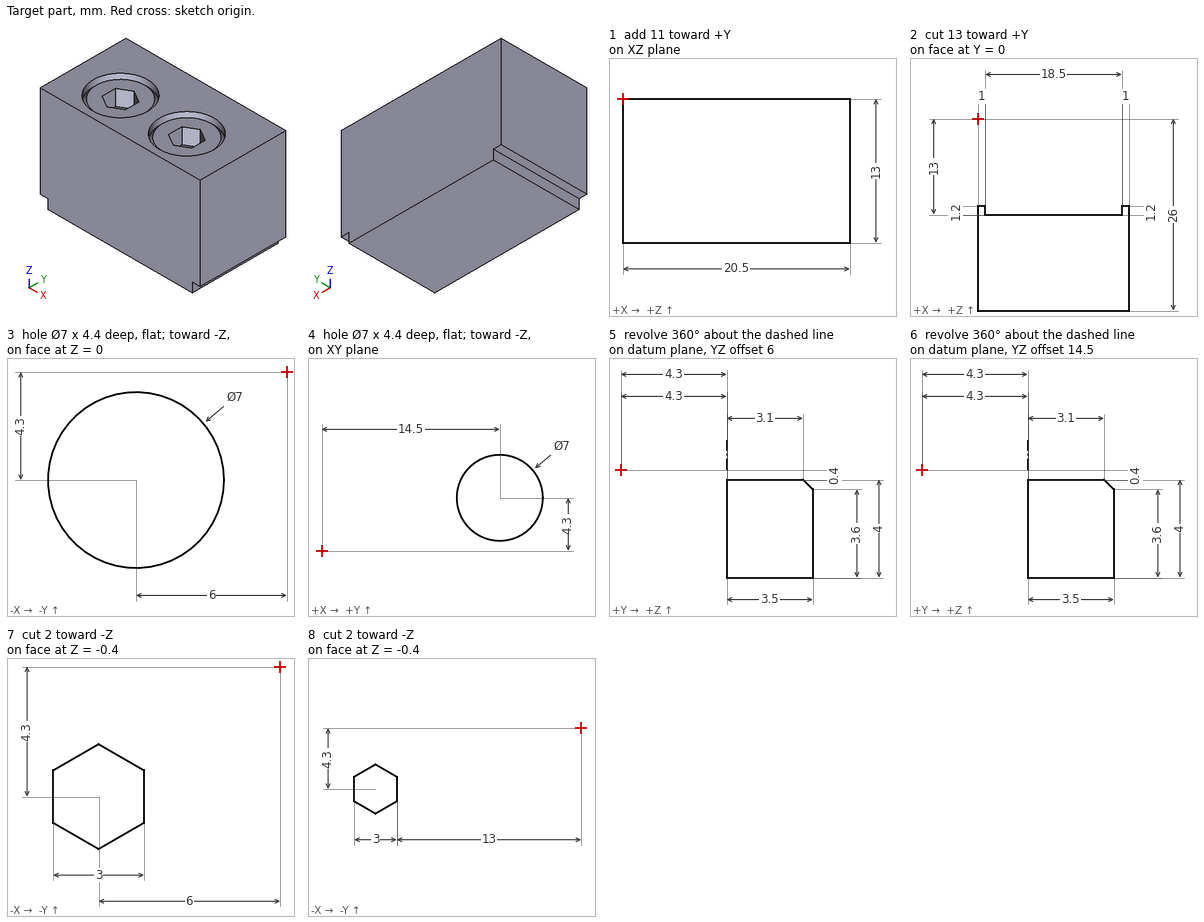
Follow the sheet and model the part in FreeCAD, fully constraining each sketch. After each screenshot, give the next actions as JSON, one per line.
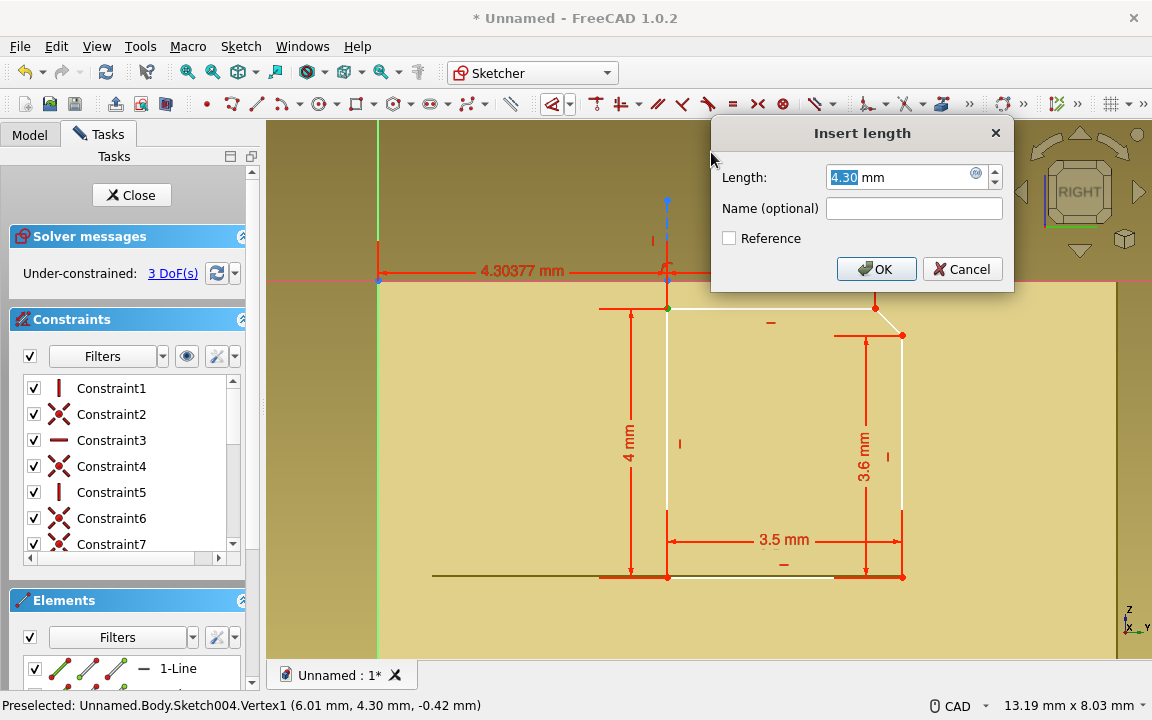
{"action": "type", "text": "4.3"}
{"action": "key", "text": "Return"}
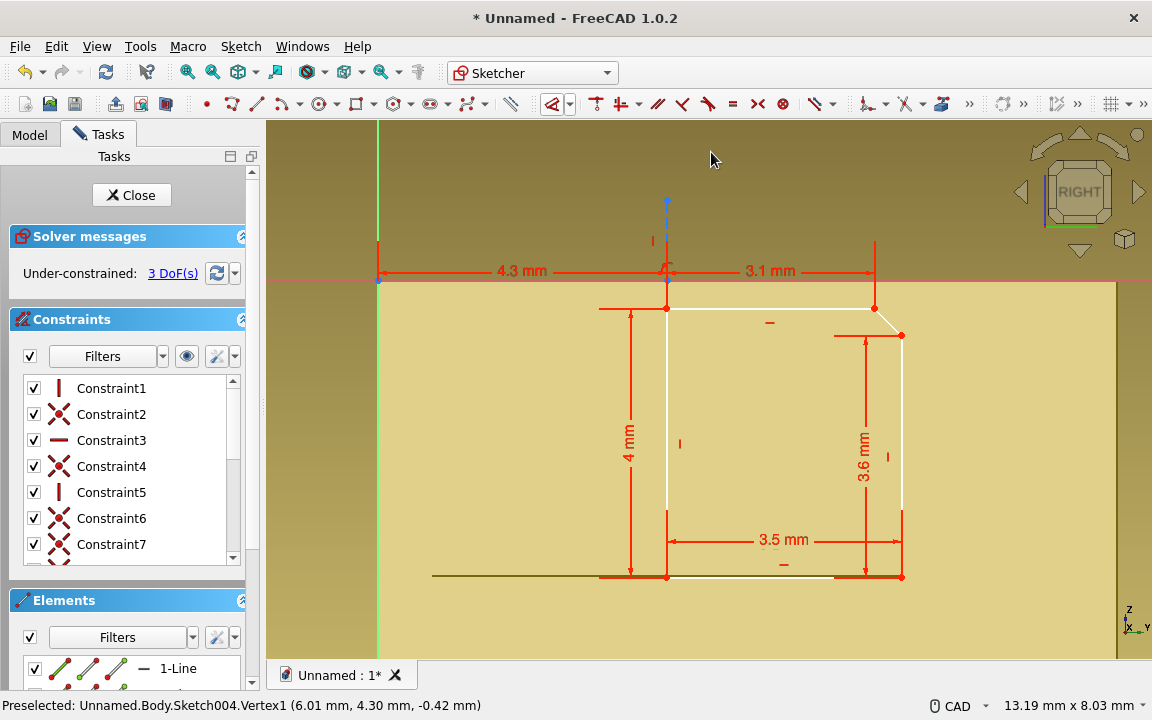
{"action": "scroll", "coordinate": [667, 309], "scroll_direction": "up", "scroll_amount": 2}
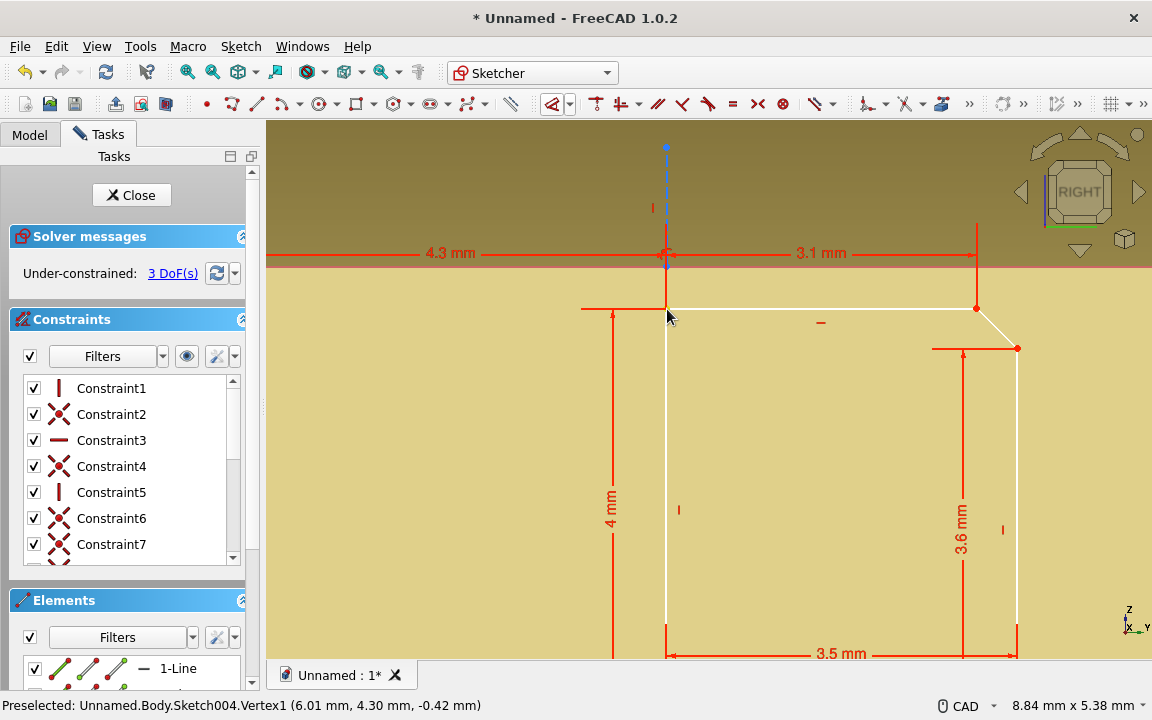
{"action": "left_click", "coordinate": [666, 309]}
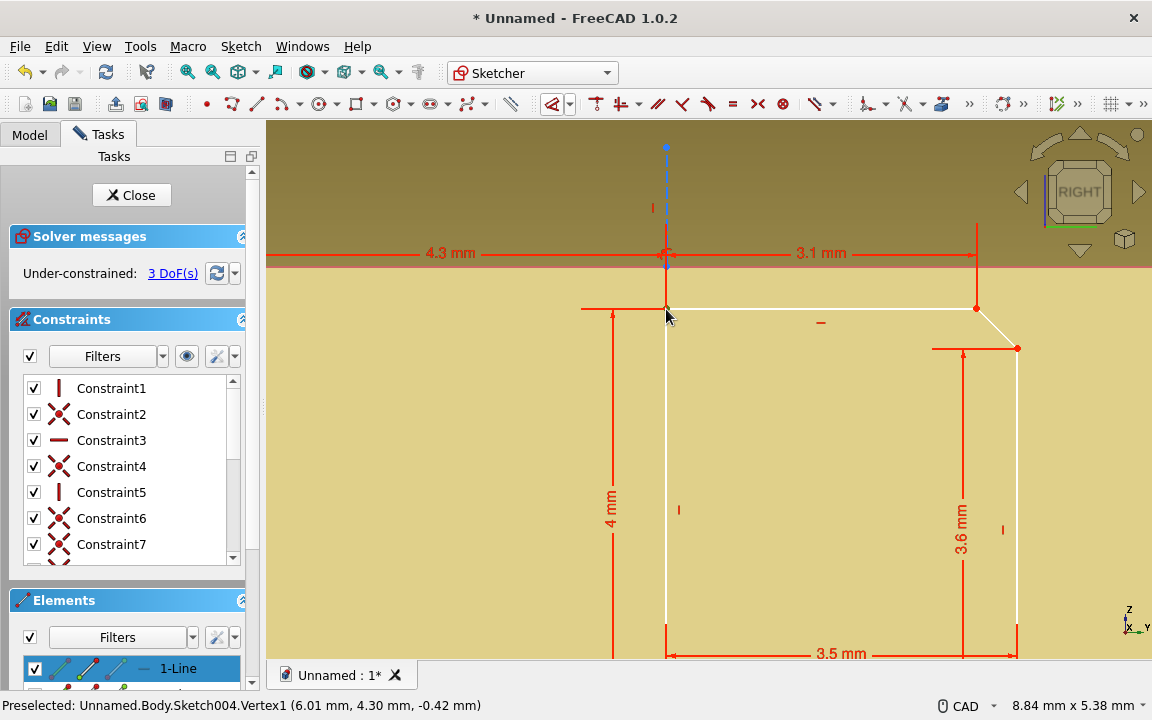
{"action": "left_click", "coordinate": [570, 104]}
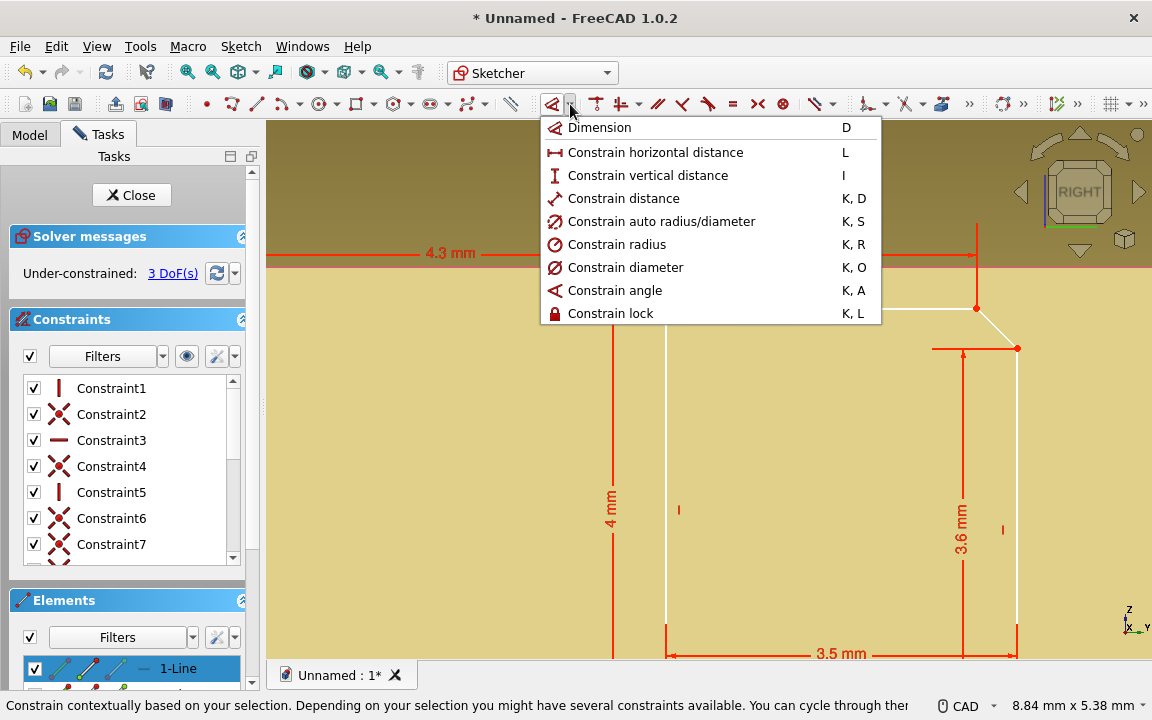
{"action": "left_click", "coordinate": [711, 176]}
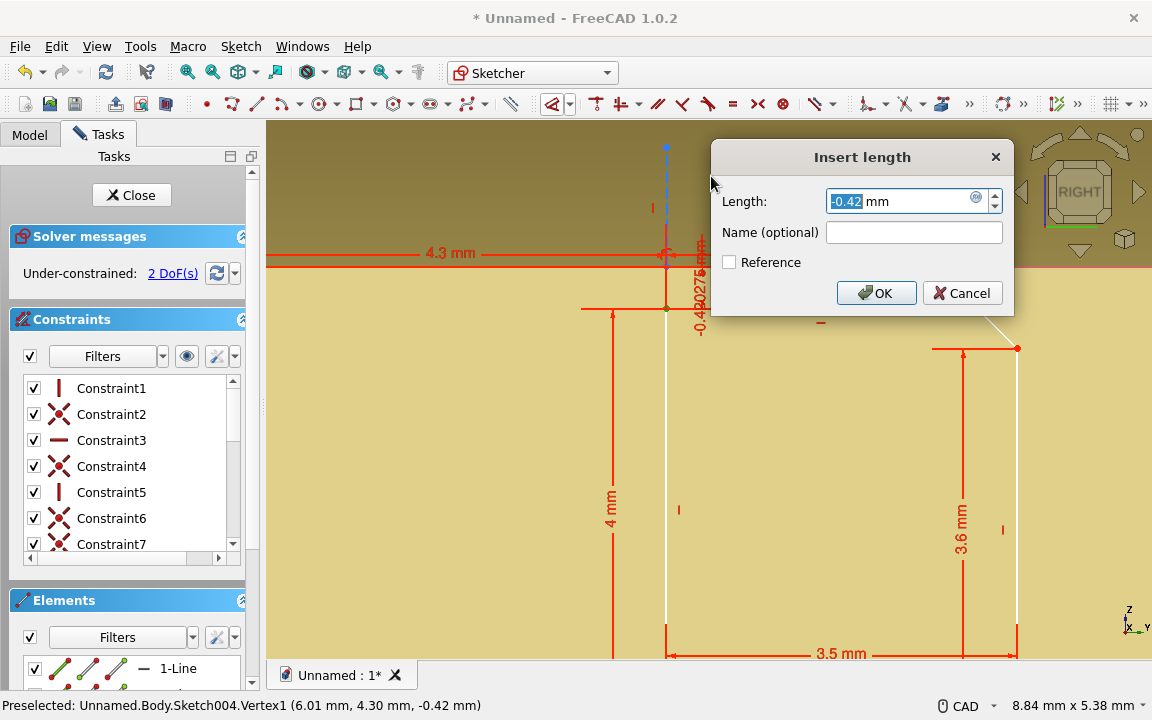
{"action": "type", "text": "-0.4"}
{"action": "key", "text": "Return"}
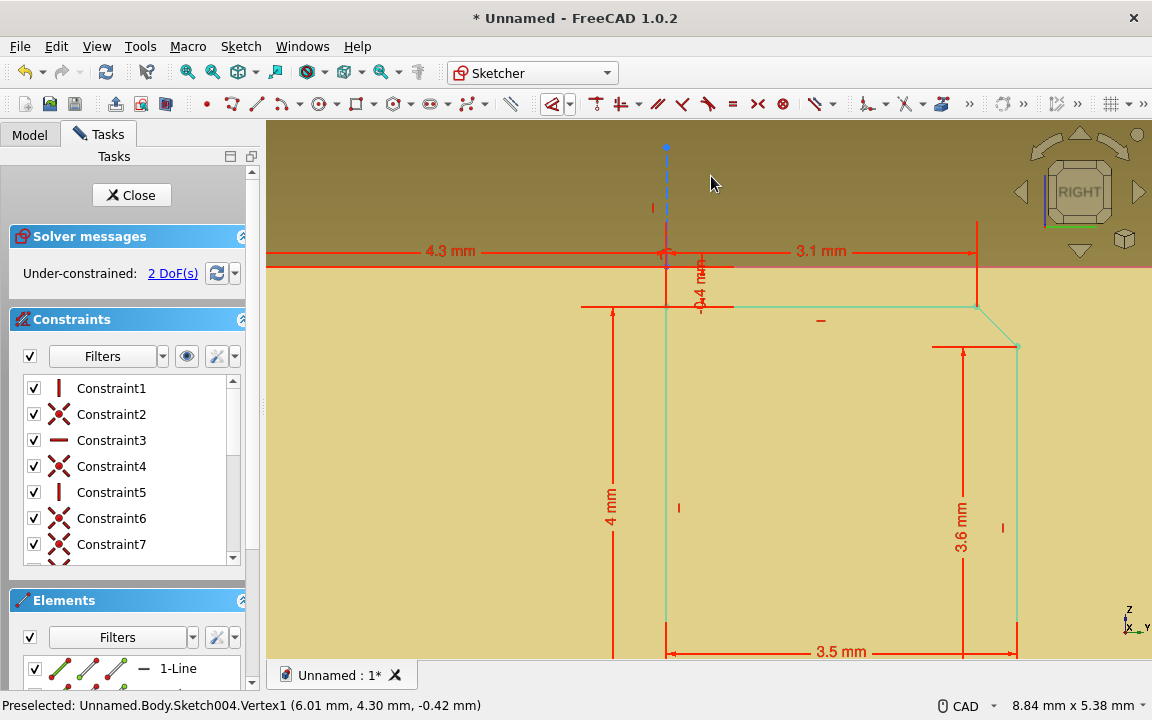
{"action": "left_click", "coordinate": [667, 267]}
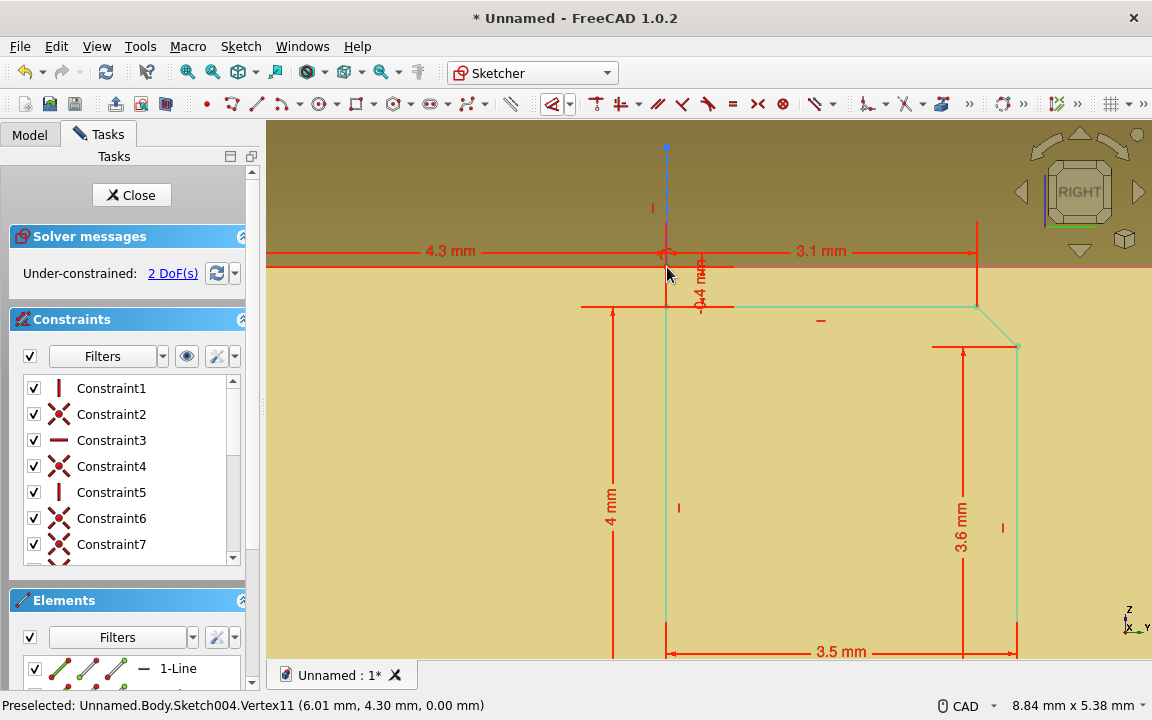
{"action": "key", "text": "l"}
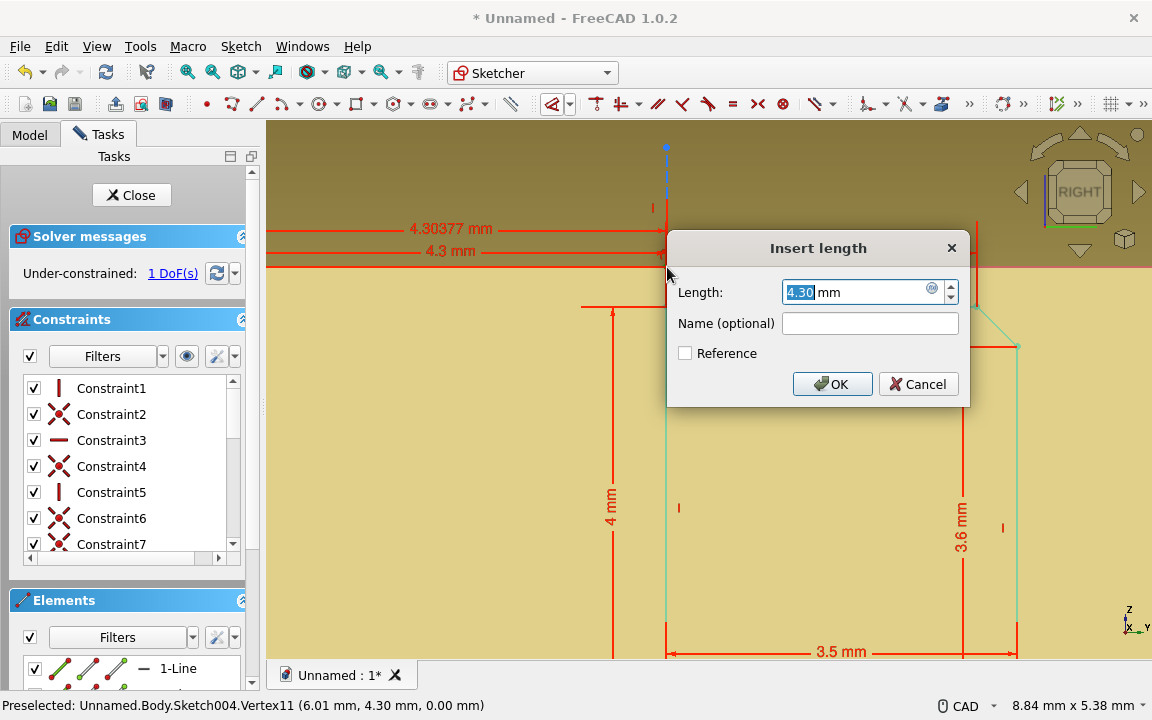
{"action": "type", "text": "4.3"}
{"action": "key", "text": "Return"}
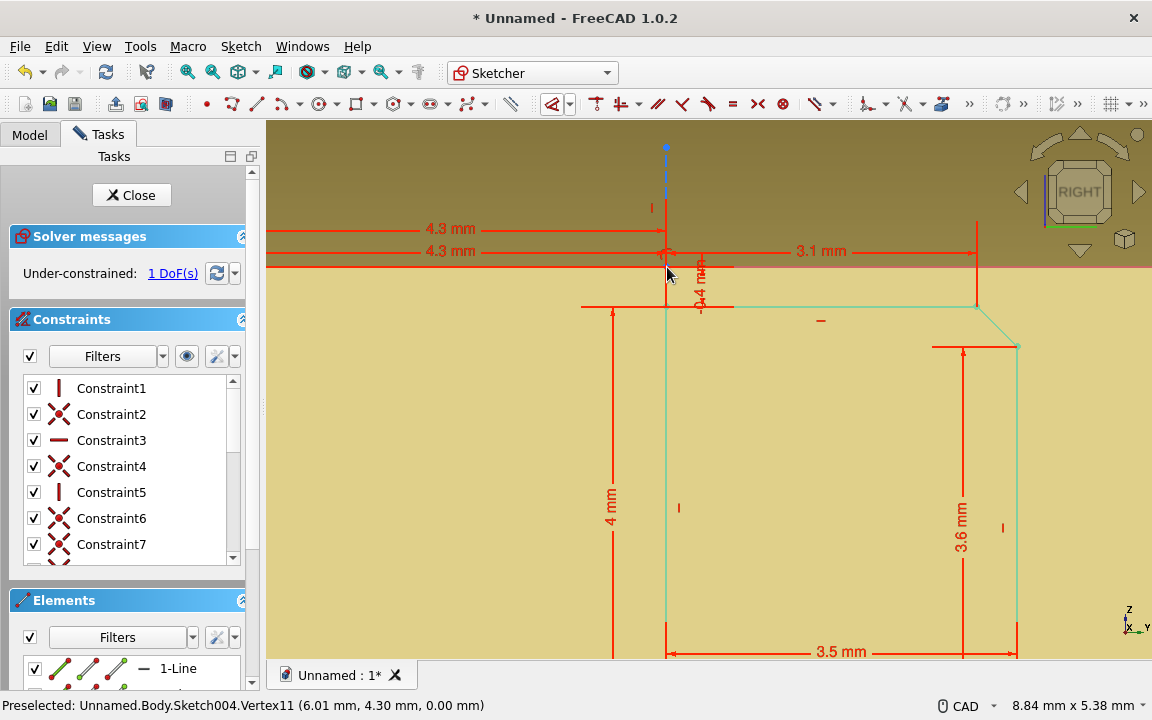
{"action": "left_click", "coordinate": [132, 195]}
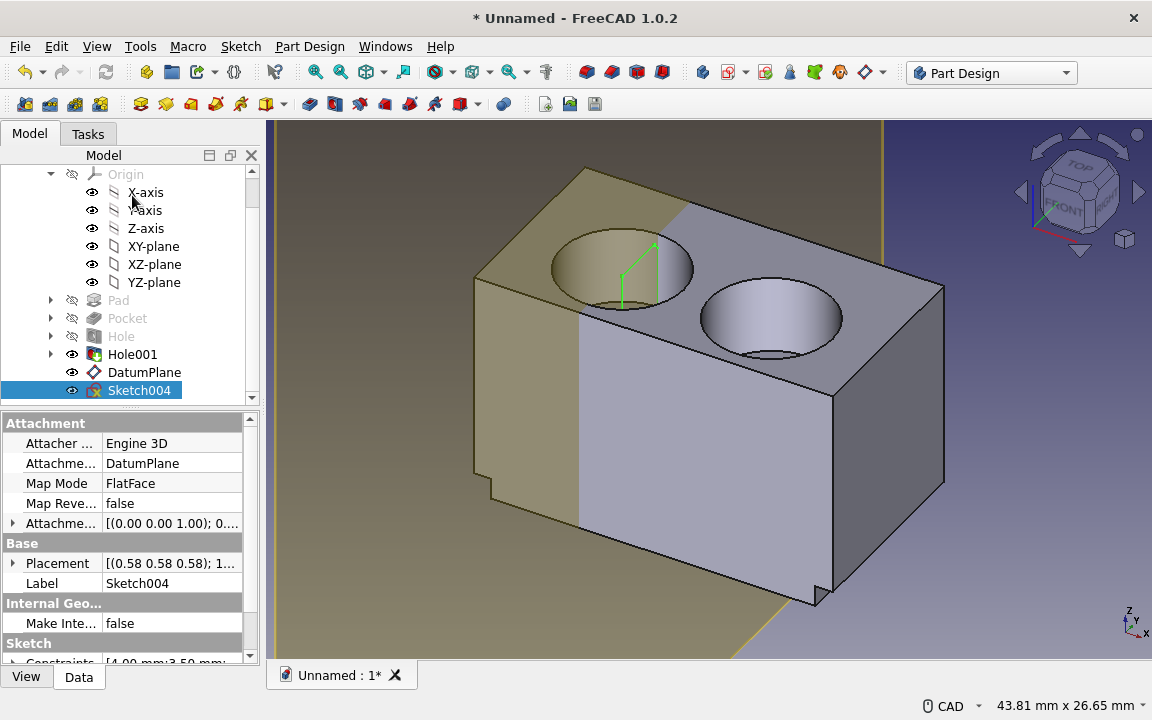
{"action": "left_click", "coordinate": [166, 104]}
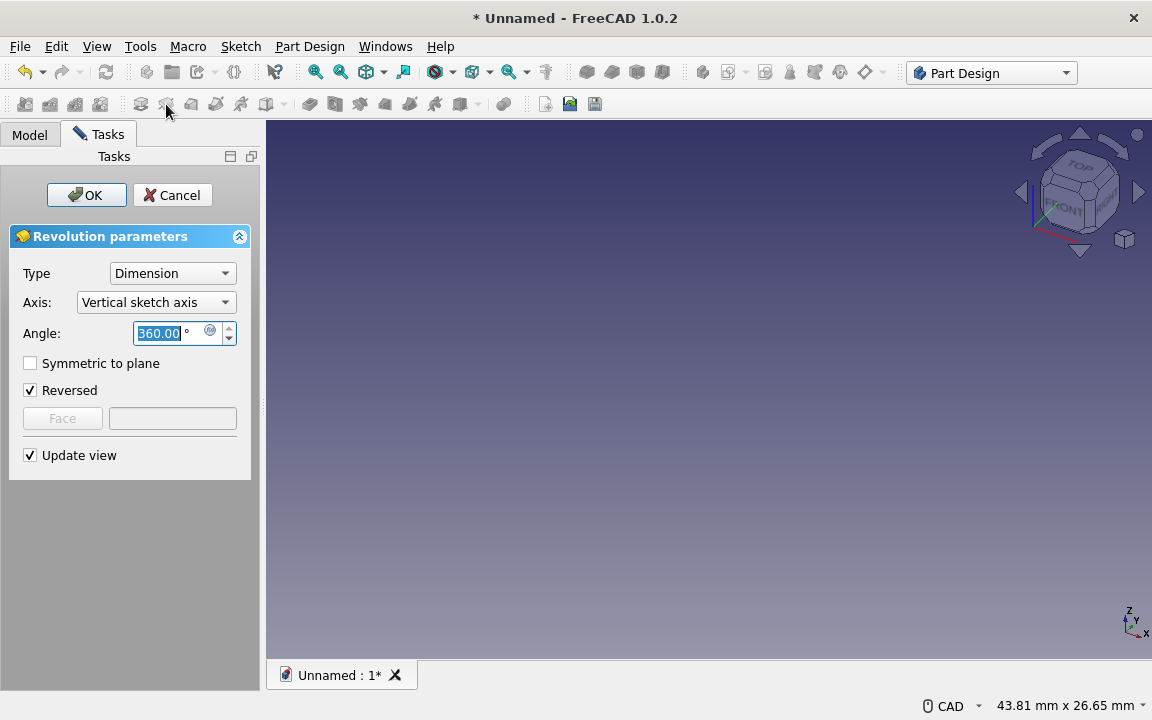
{"action": "left_click", "coordinate": [157, 302]}